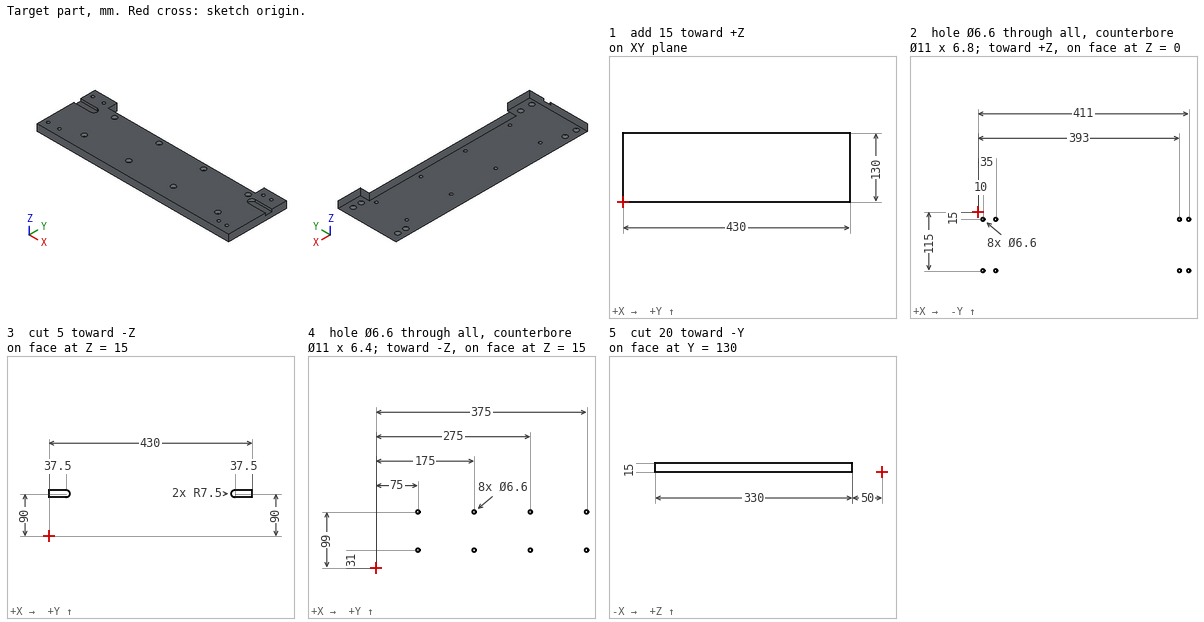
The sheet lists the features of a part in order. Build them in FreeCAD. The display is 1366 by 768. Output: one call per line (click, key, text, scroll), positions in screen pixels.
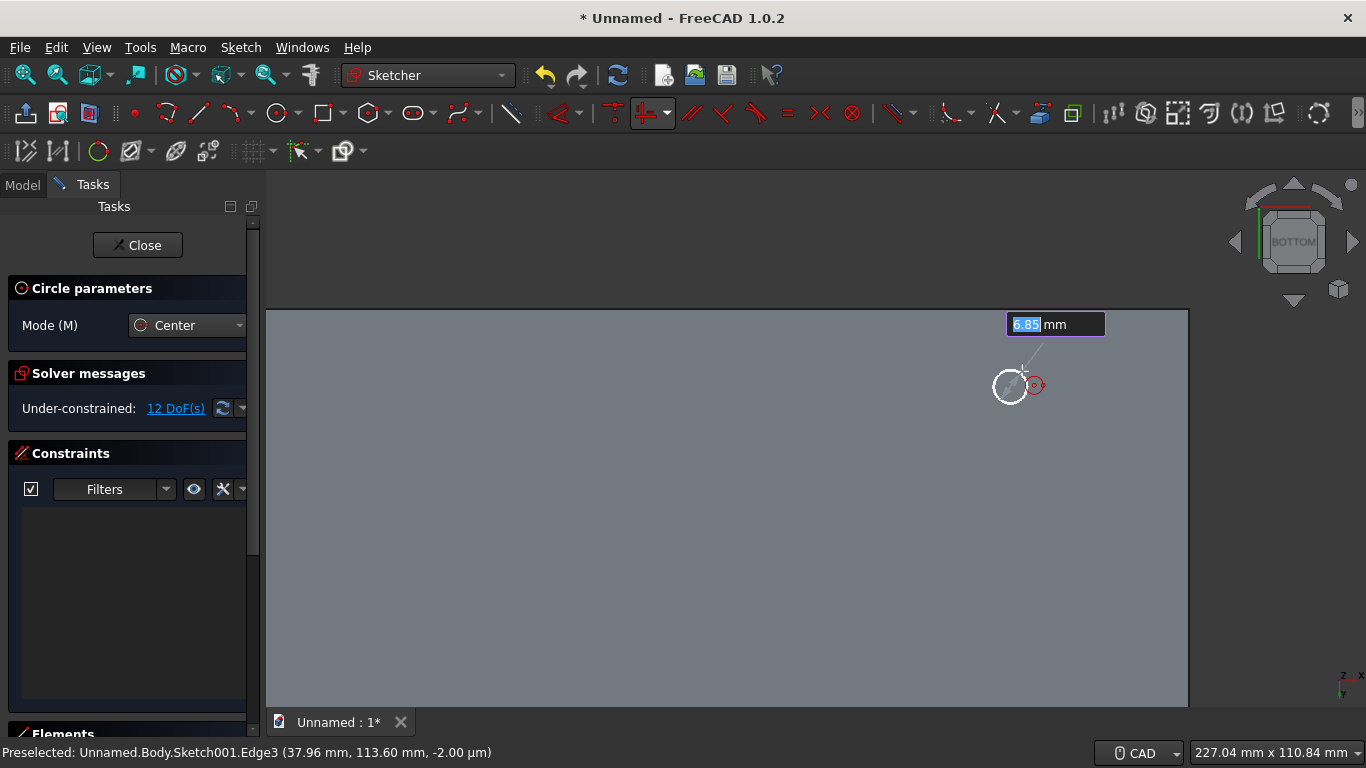
click(1021, 371)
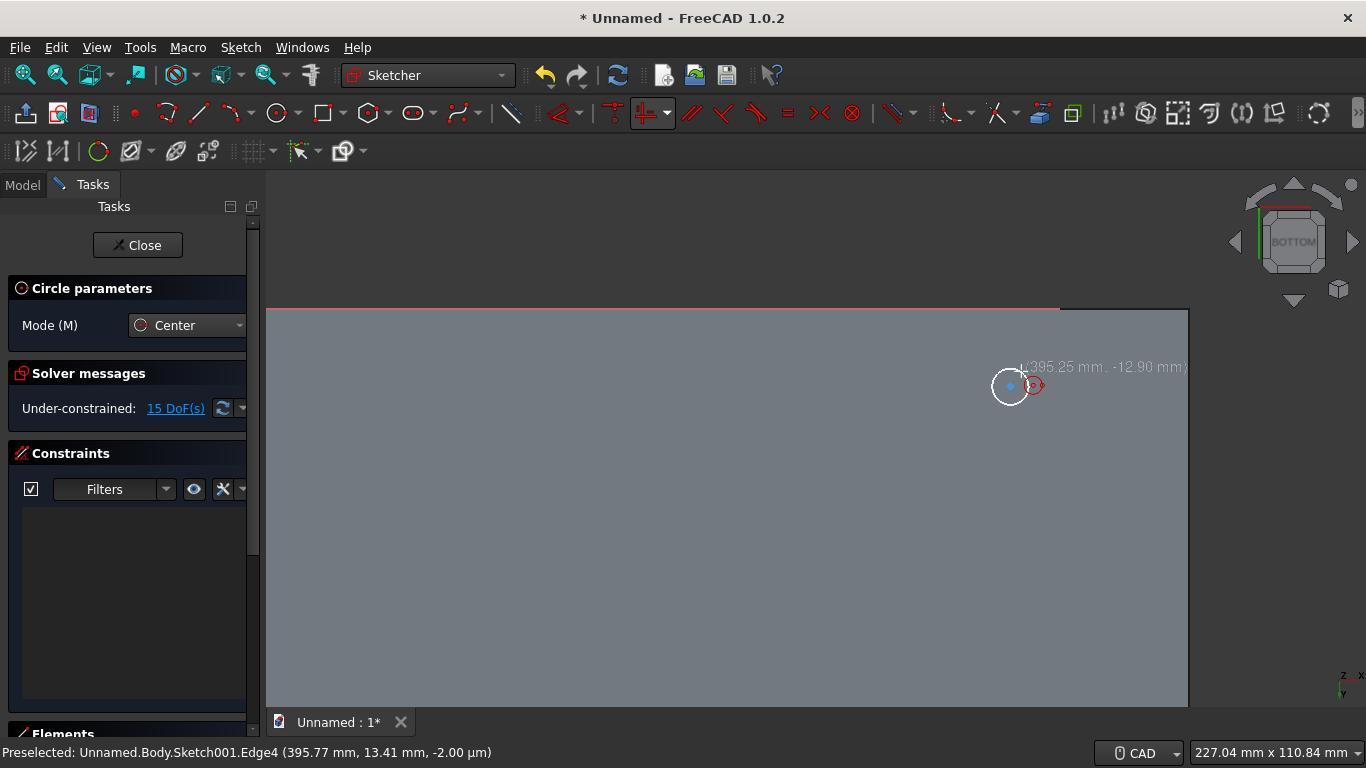
scroll(1097, 382, up, 2)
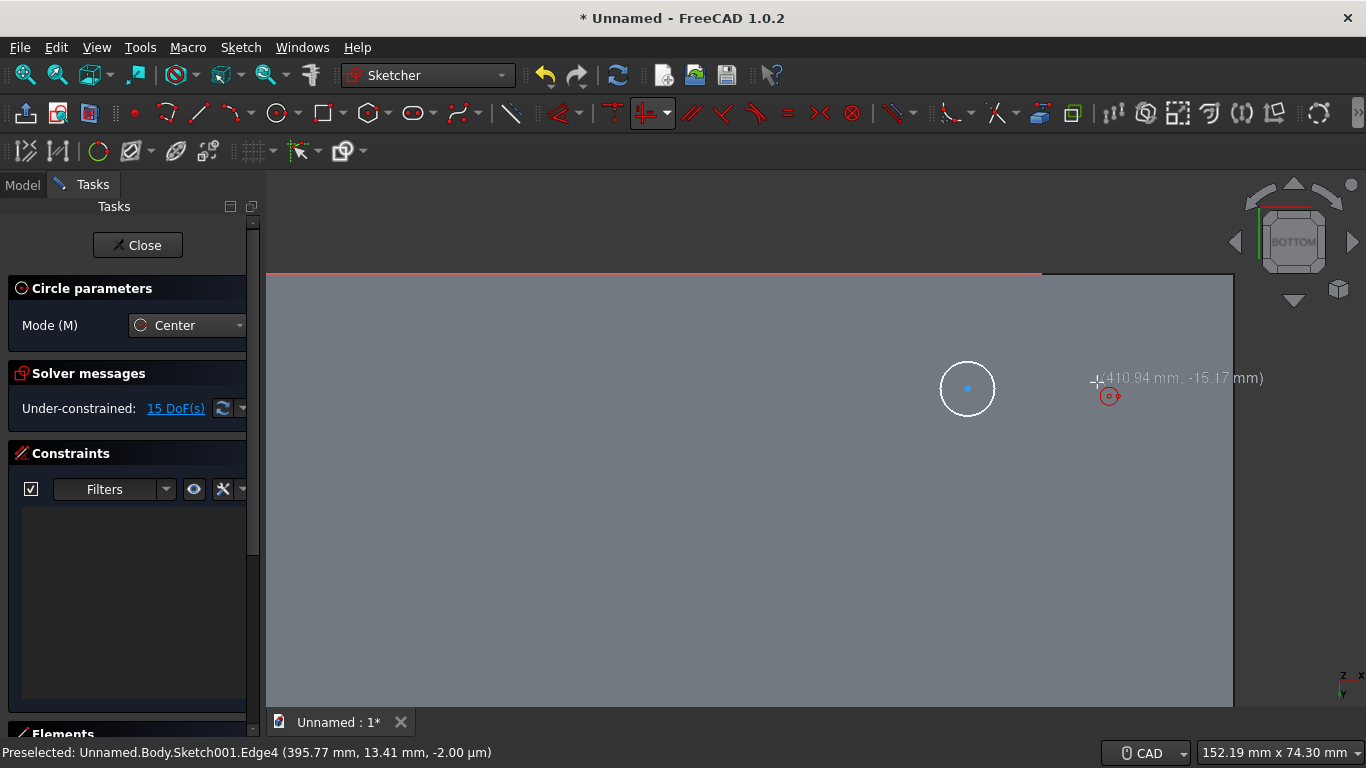
scroll(1032, 372, down, 8)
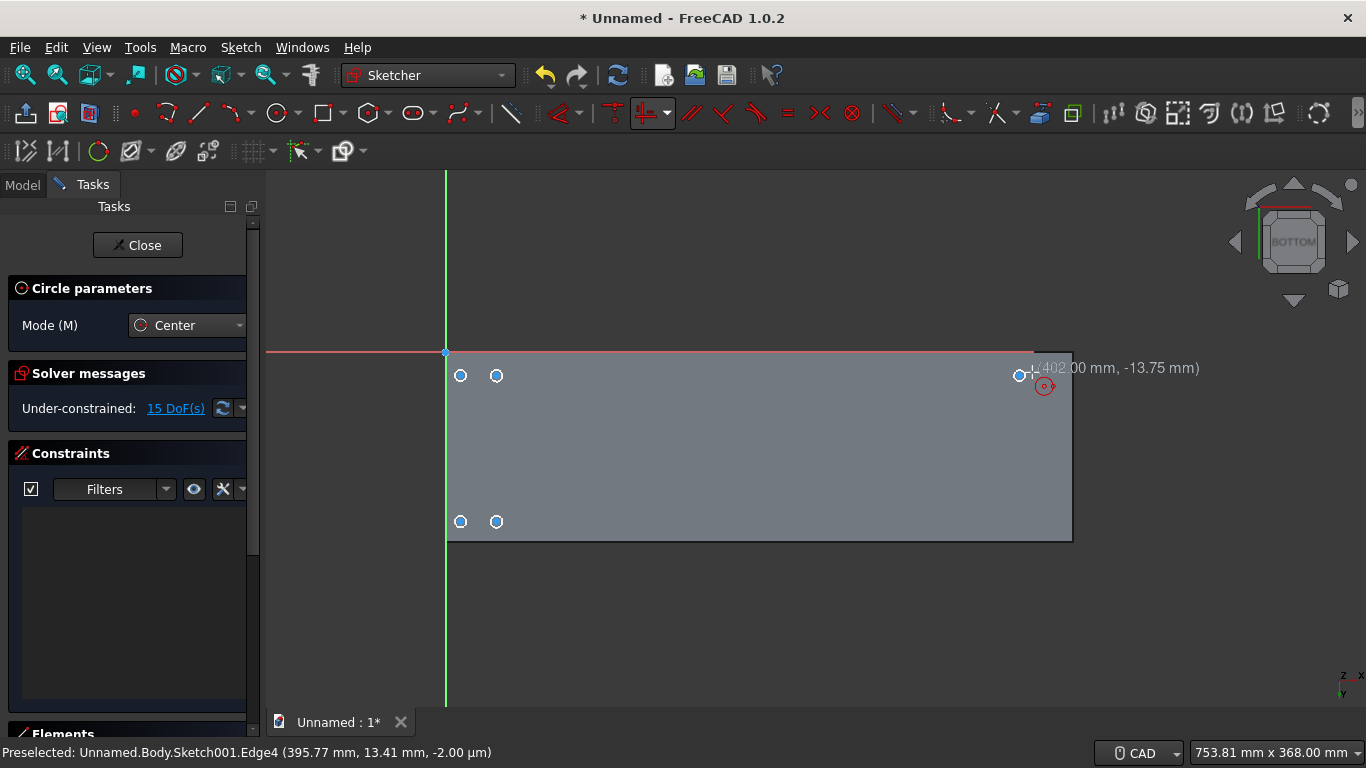
click(1046, 374)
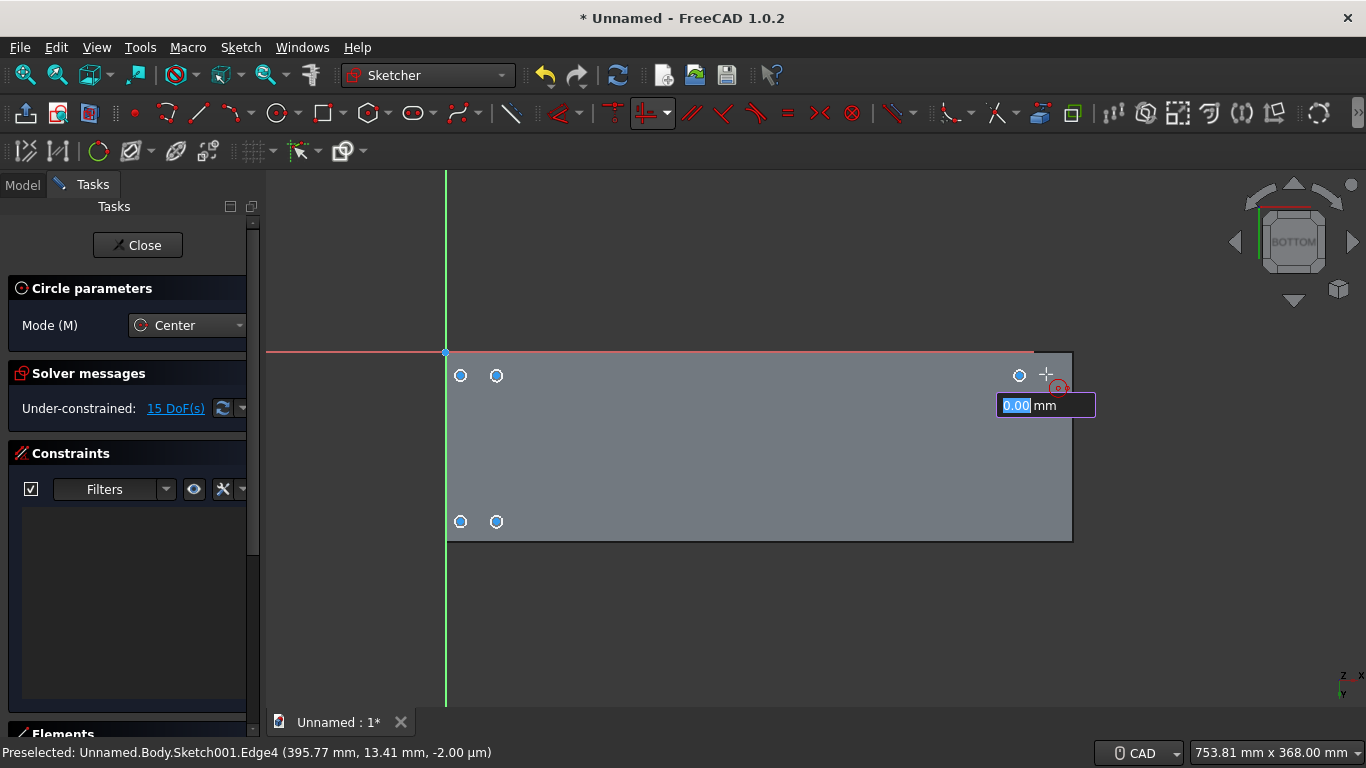
scroll(1049, 371, up, 6)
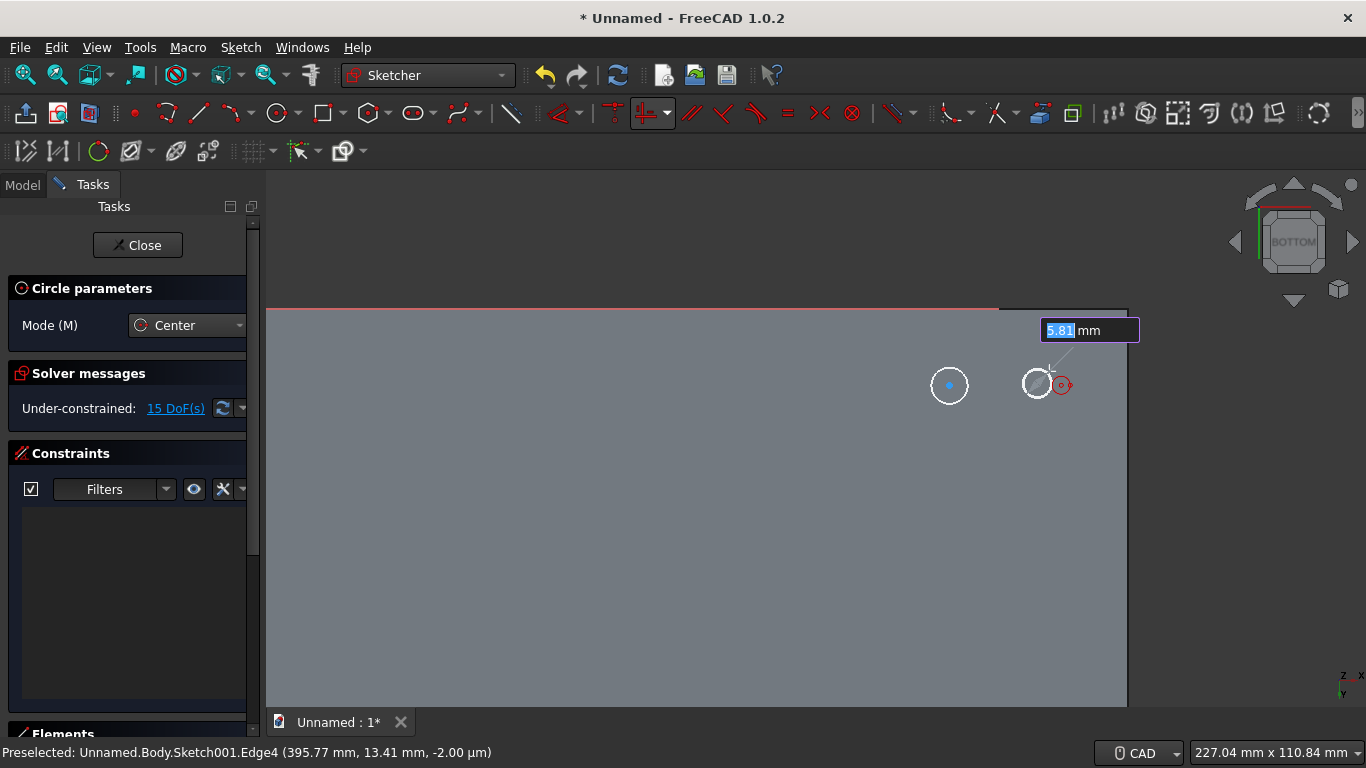
click(1048, 370)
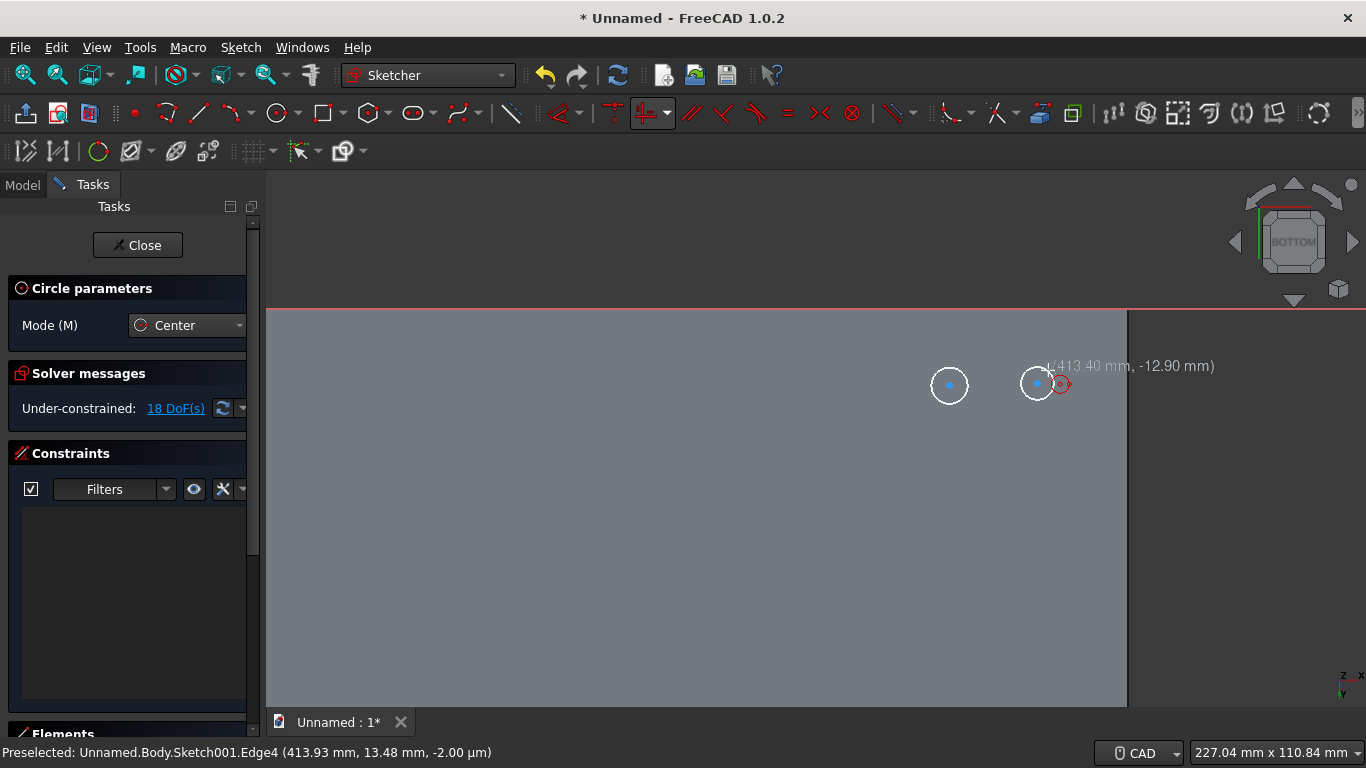
scroll(1049, 371, down, 6)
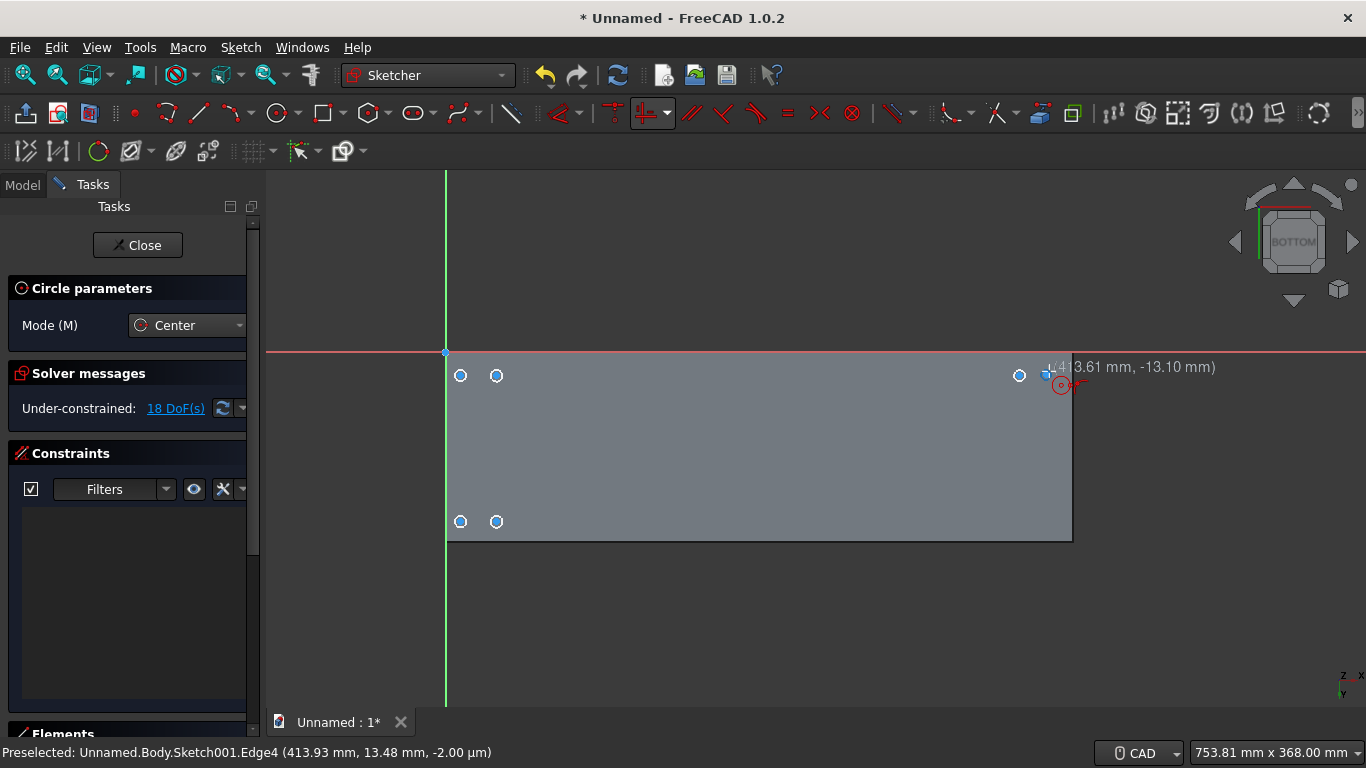
scroll(1019, 520, up, 8)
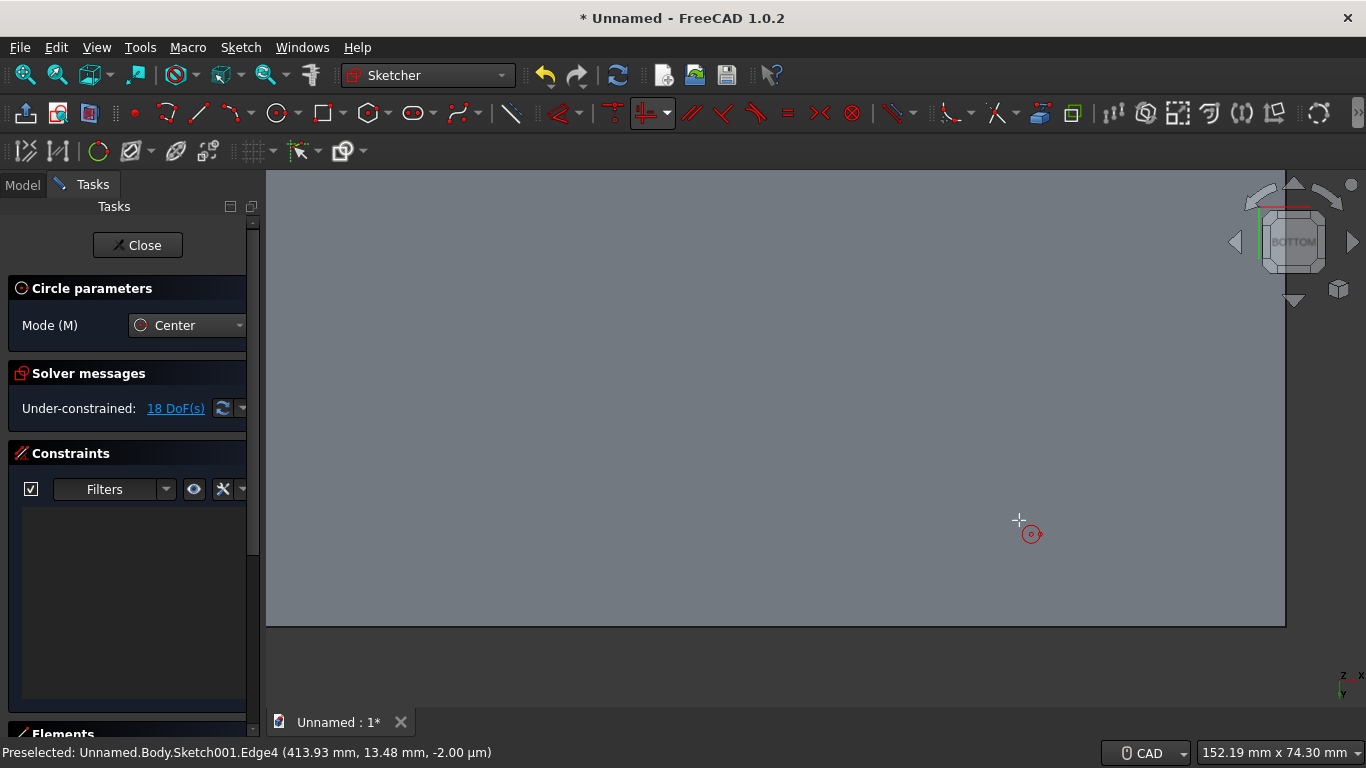
scroll(1019, 520, down, 8)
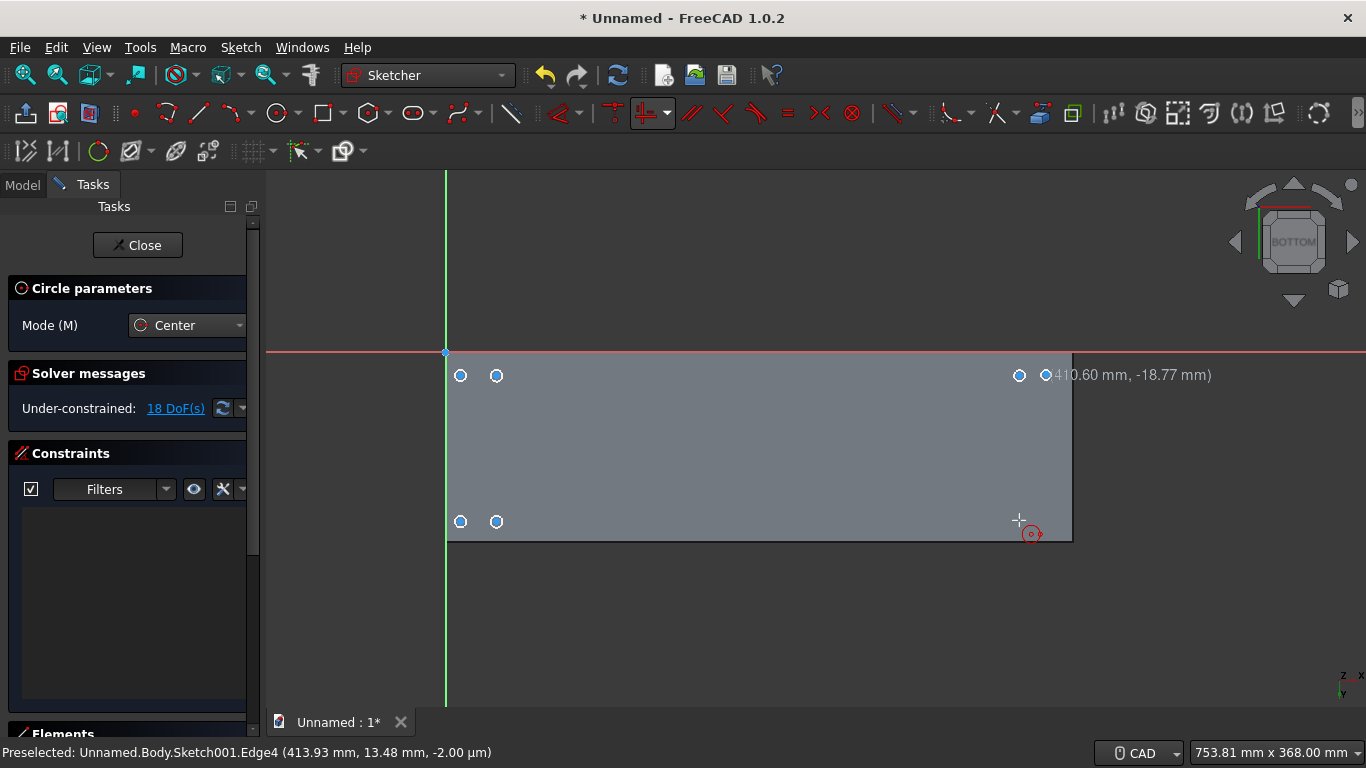
click(1019, 520)